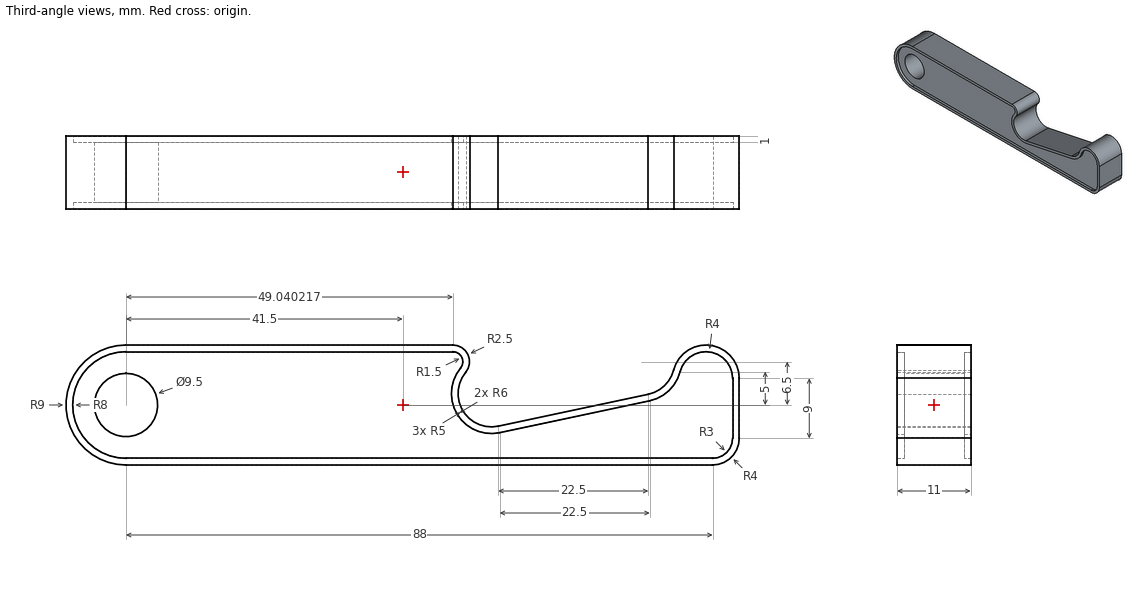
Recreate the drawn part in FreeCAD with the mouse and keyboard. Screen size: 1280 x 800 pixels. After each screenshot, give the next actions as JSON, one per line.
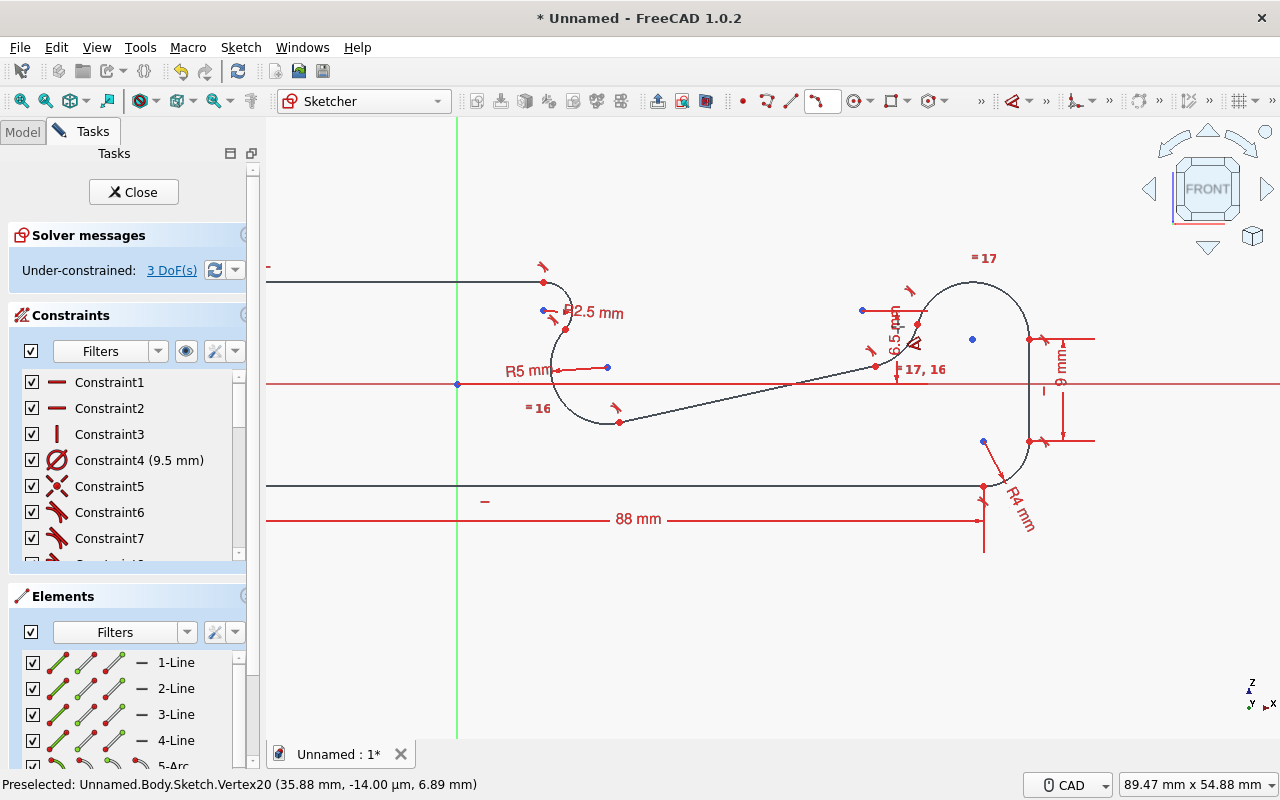
{"action": "scroll", "coordinate": [1005, 481], "scroll_direction": "down", "scroll_amount": 3}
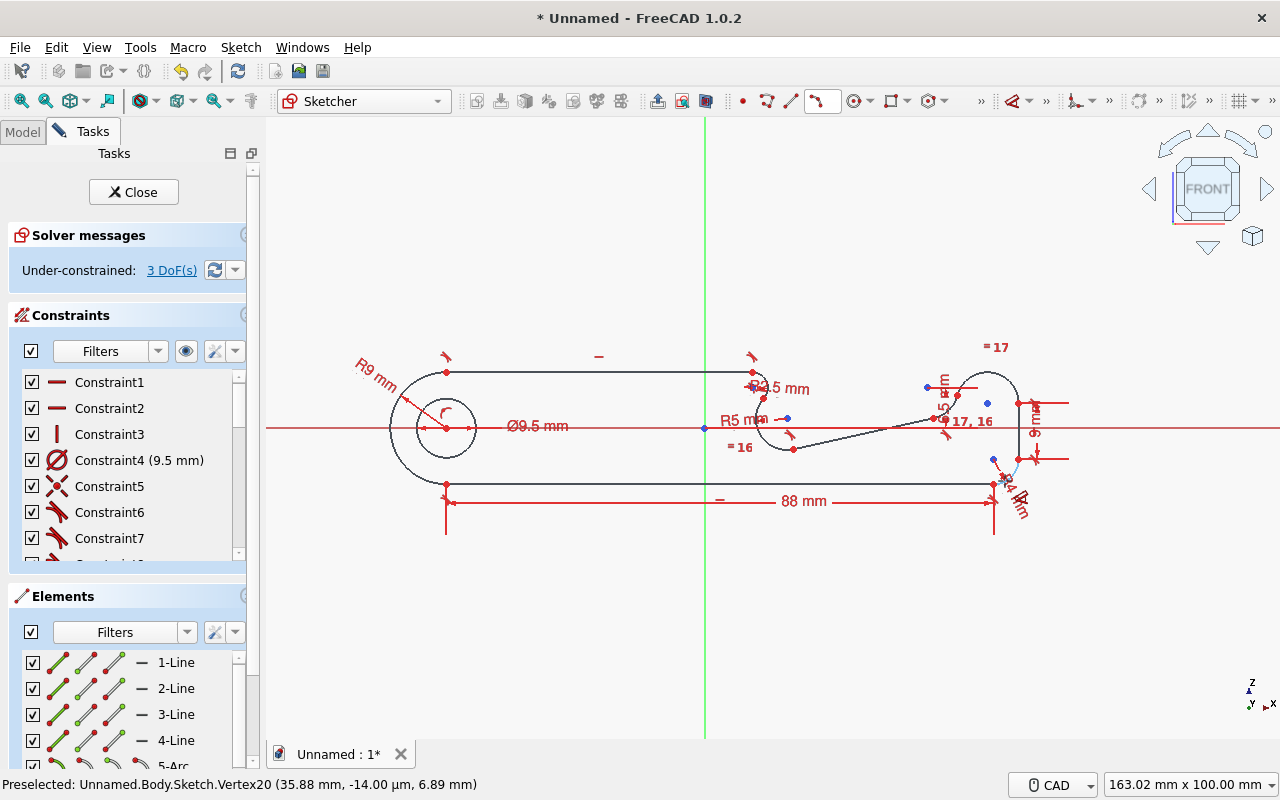
{"action": "left_click", "coordinate": [446, 428]}
{"action": "left_click", "coordinate": [576, 462]}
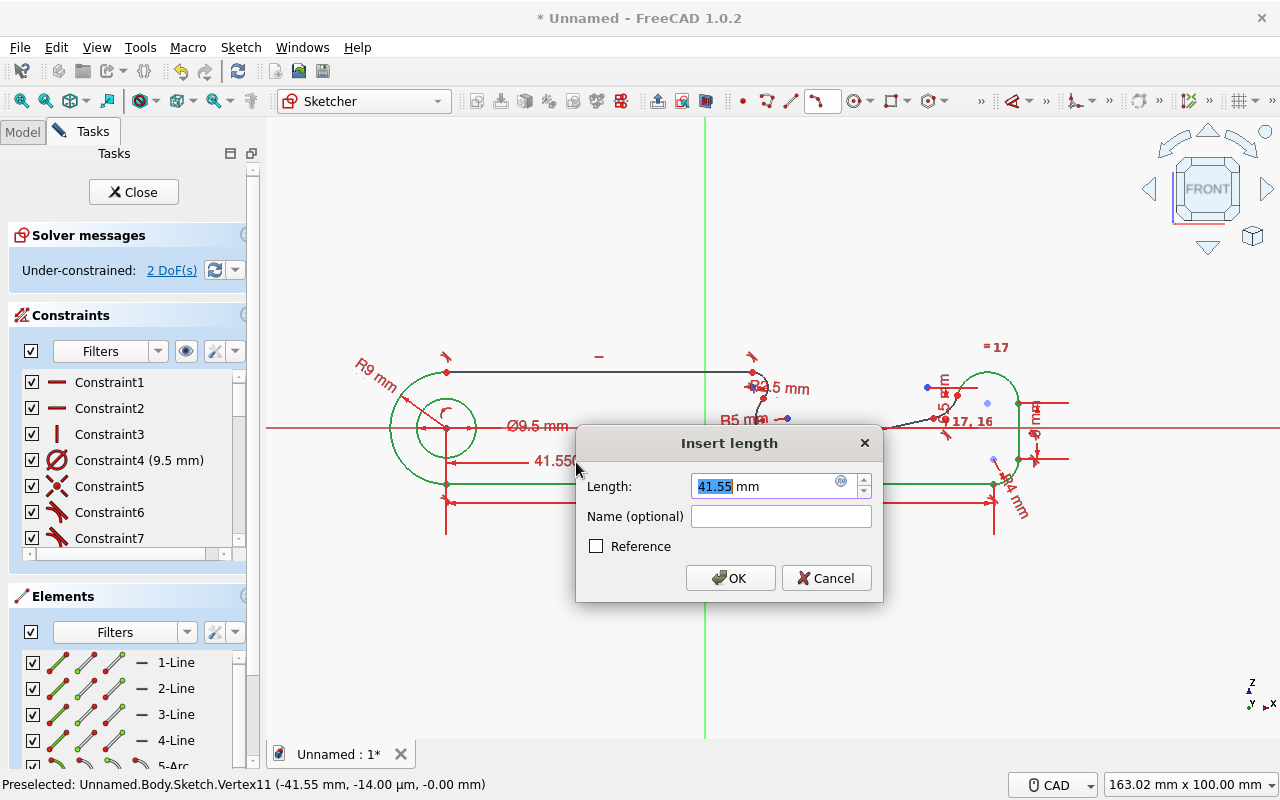
{"action": "type", "text": "41.5"}
{"action": "key", "text": "Return"}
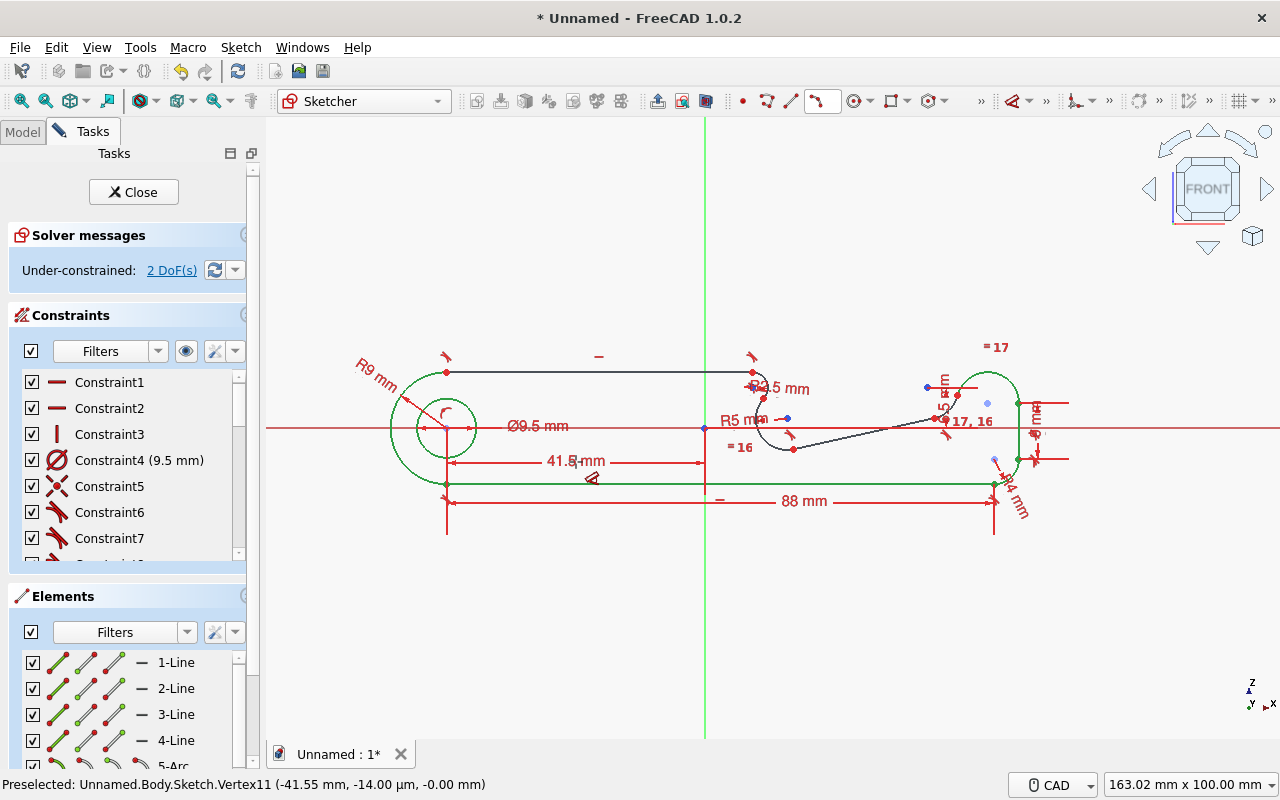
{"action": "left_click", "coordinate": [836, 440]}
{"action": "left_click", "coordinate": [864, 384]}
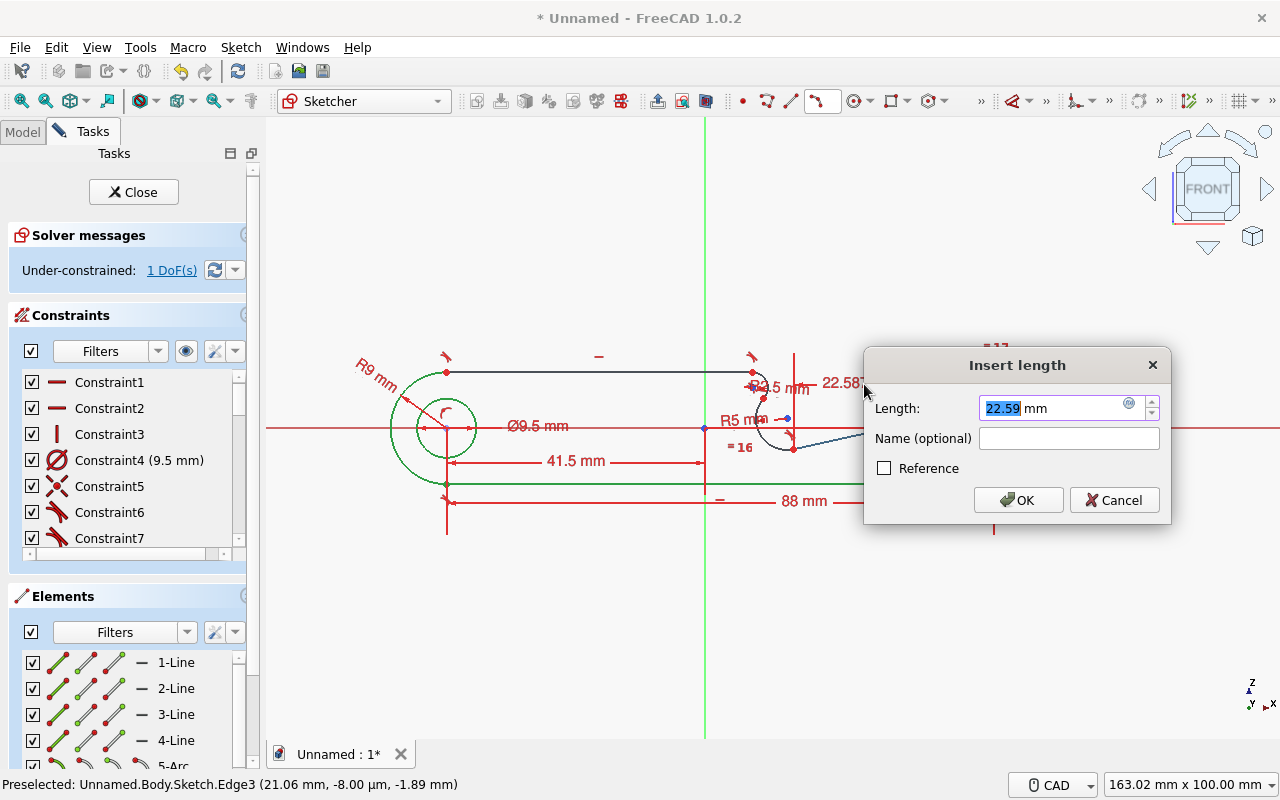
{"action": "type", "text": "22.5"}
{"action": "key", "text": "Return"}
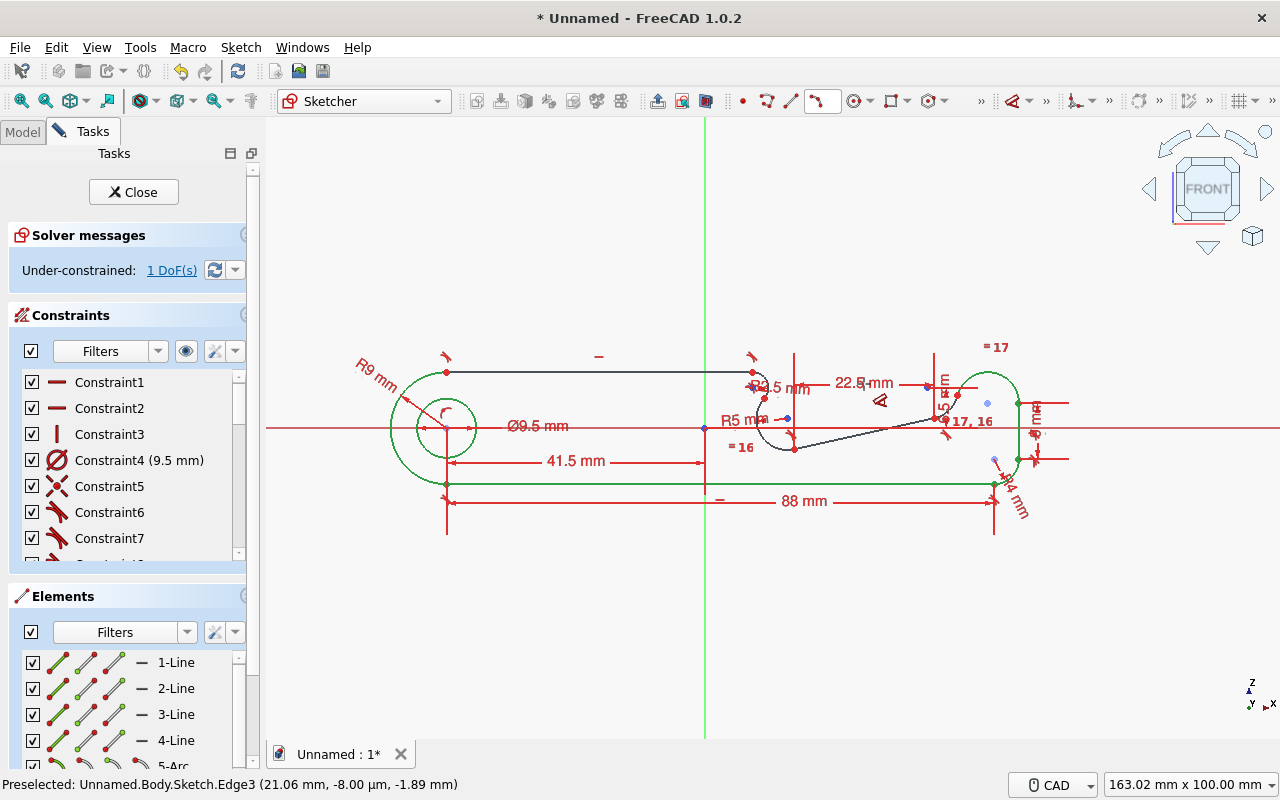
{"action": "left_click", "coordinate": [539, 372]}
{"action": "left_click", "coordinate": [600, 338]}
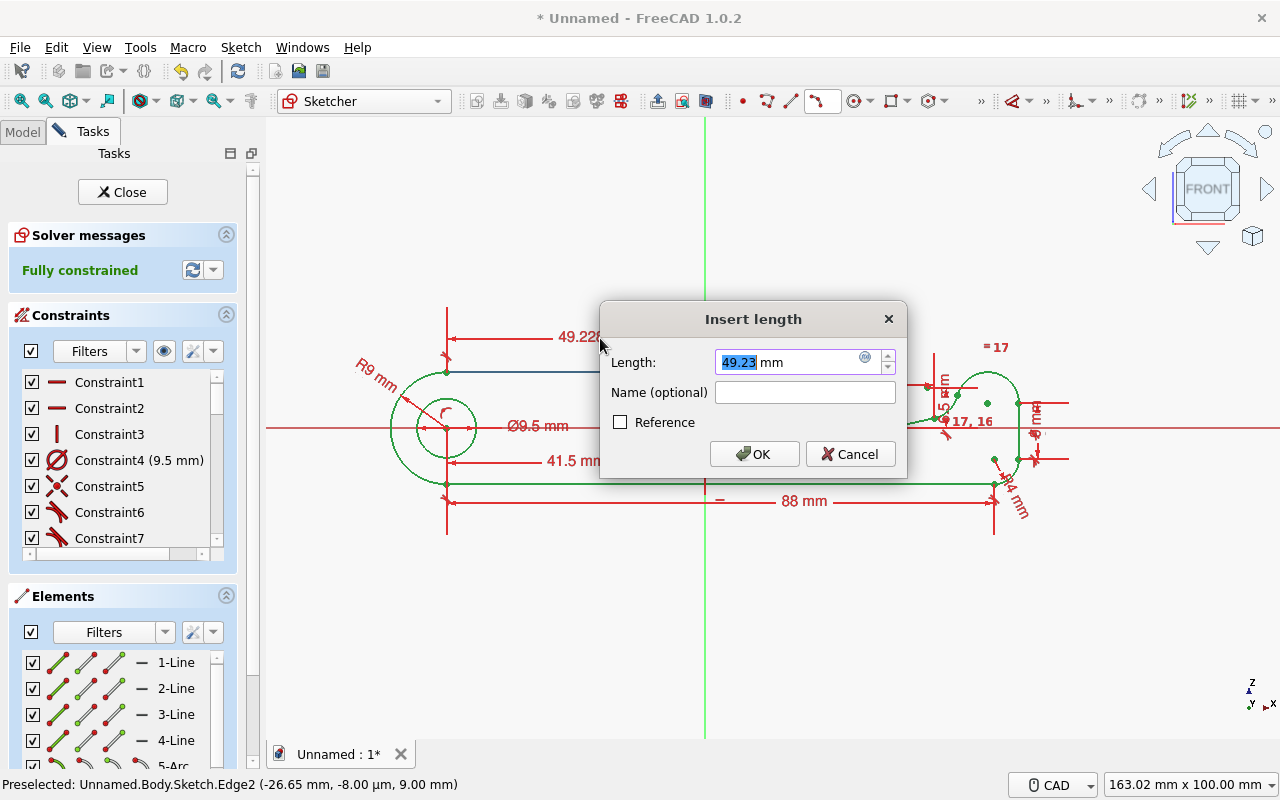
{"action": "type", "text": "49.040217"}
{"action": "key", "text": "Return"}
{"action": "key", "text": "Escape"}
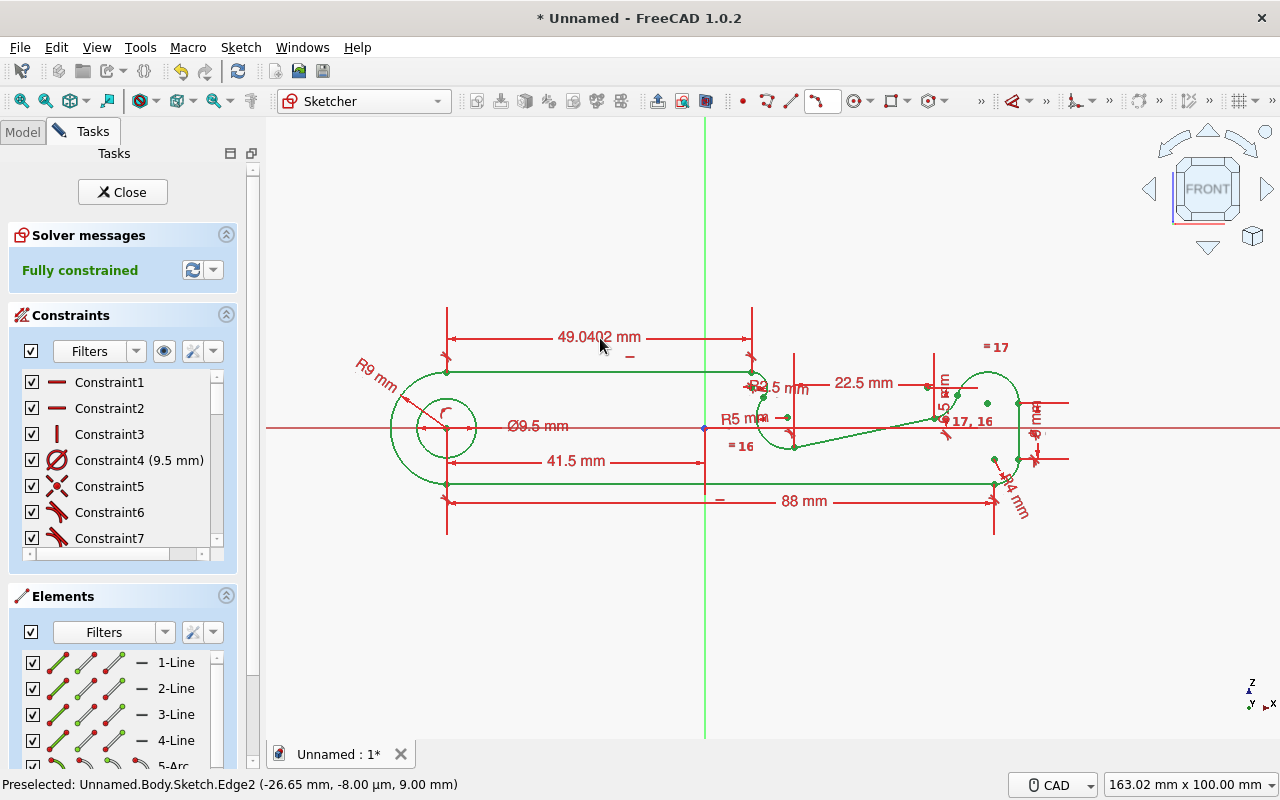
{"action": "left_click", "coordinate": [123, 192]}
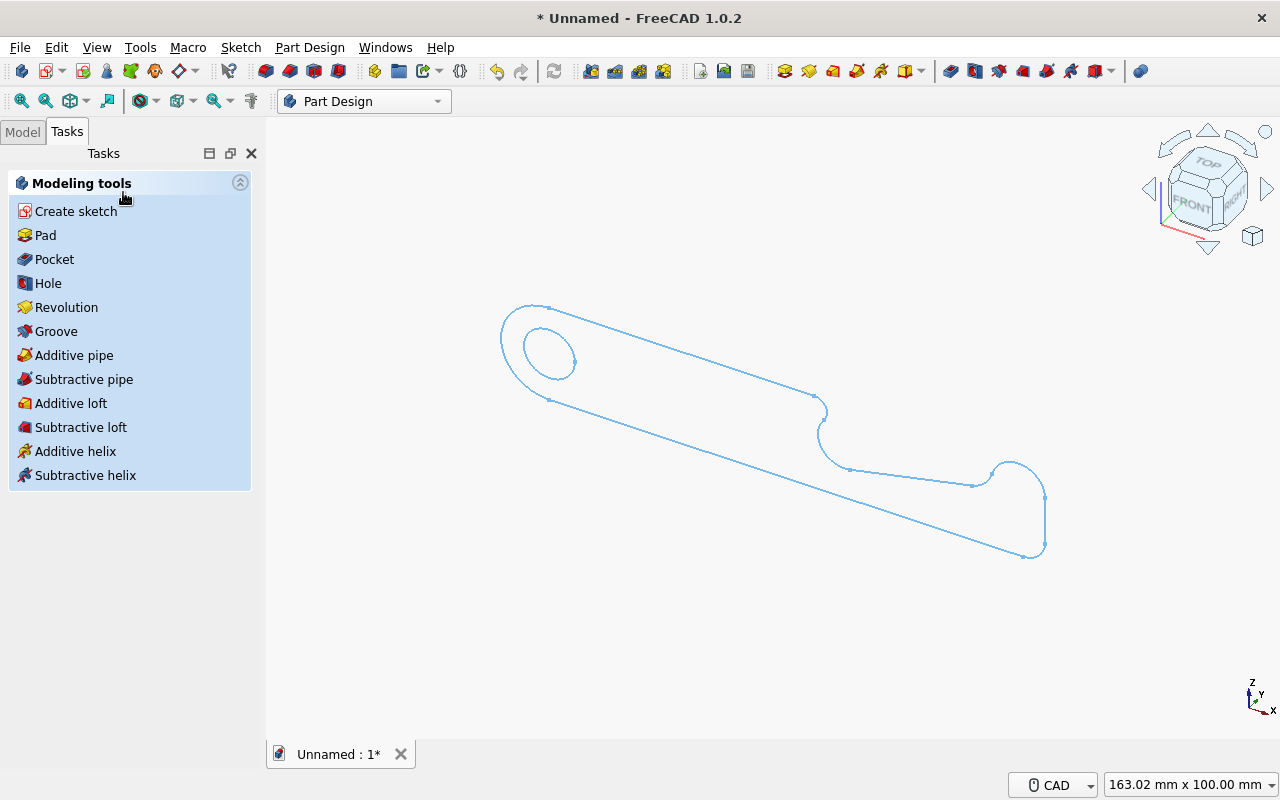
{"action": "left_click", "coordinate": [786, 72]}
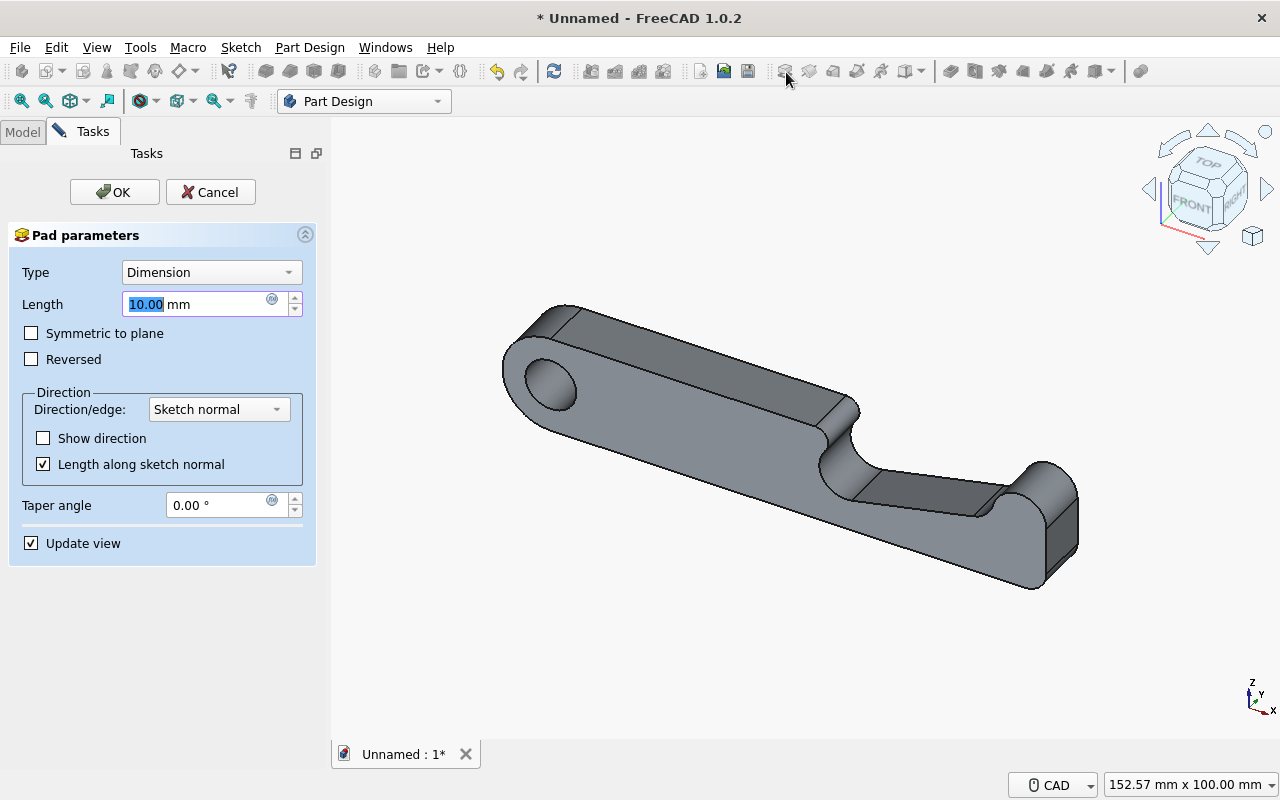
{"action": "type", "text": "11"}
{"action": "key", "text": "Tab"}